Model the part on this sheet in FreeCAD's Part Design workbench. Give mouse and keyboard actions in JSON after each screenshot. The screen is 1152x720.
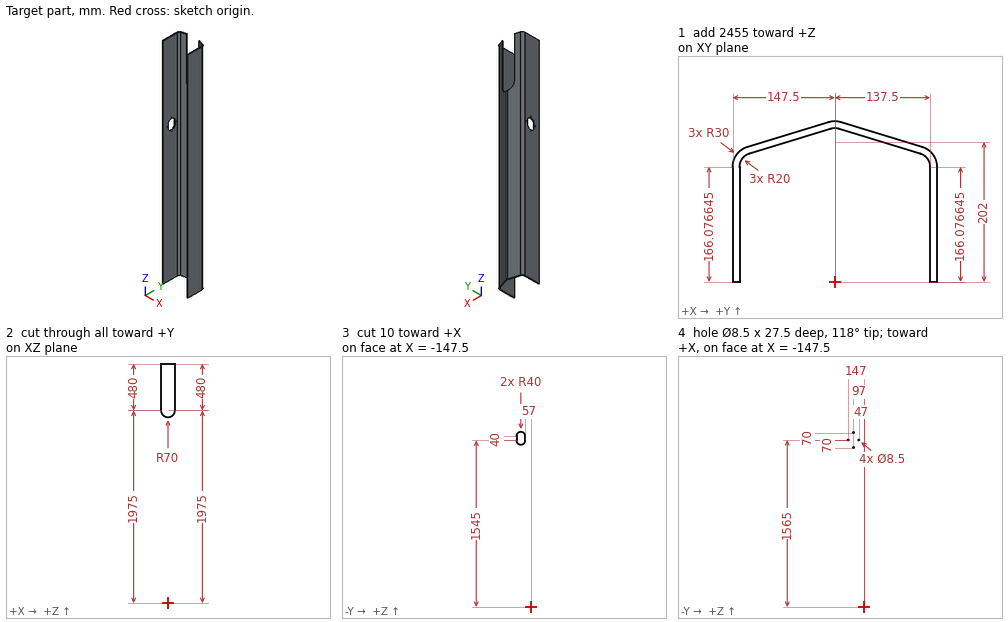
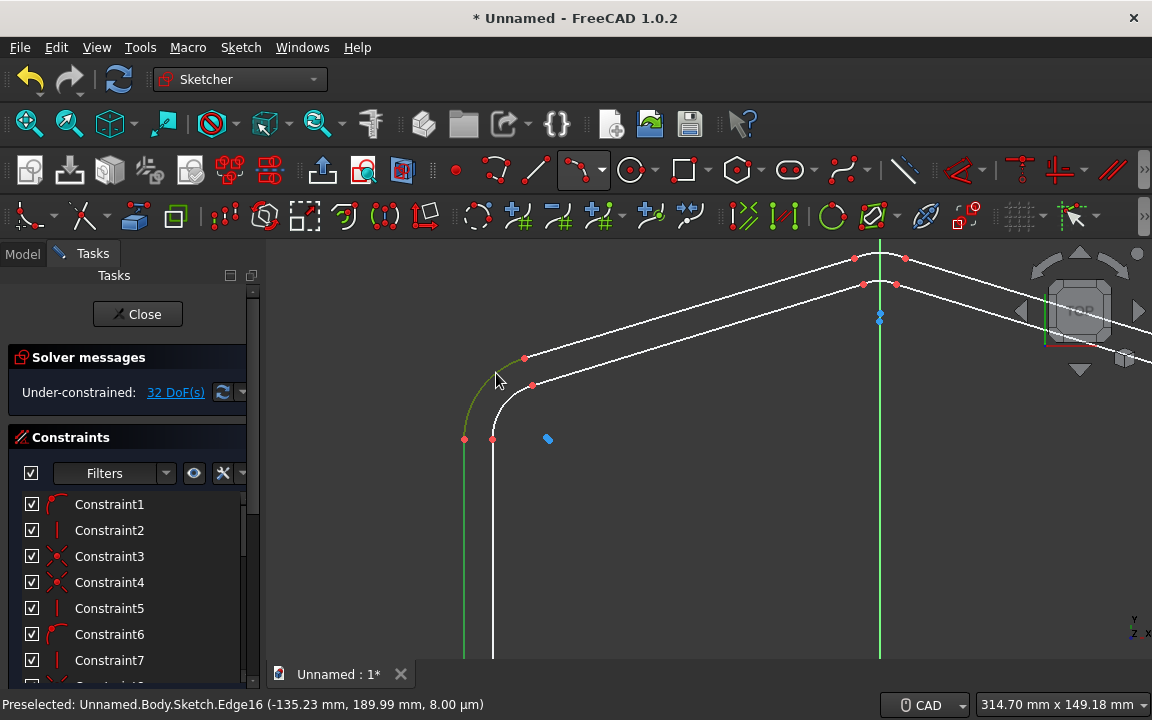
{"action": "key", "text": "t"}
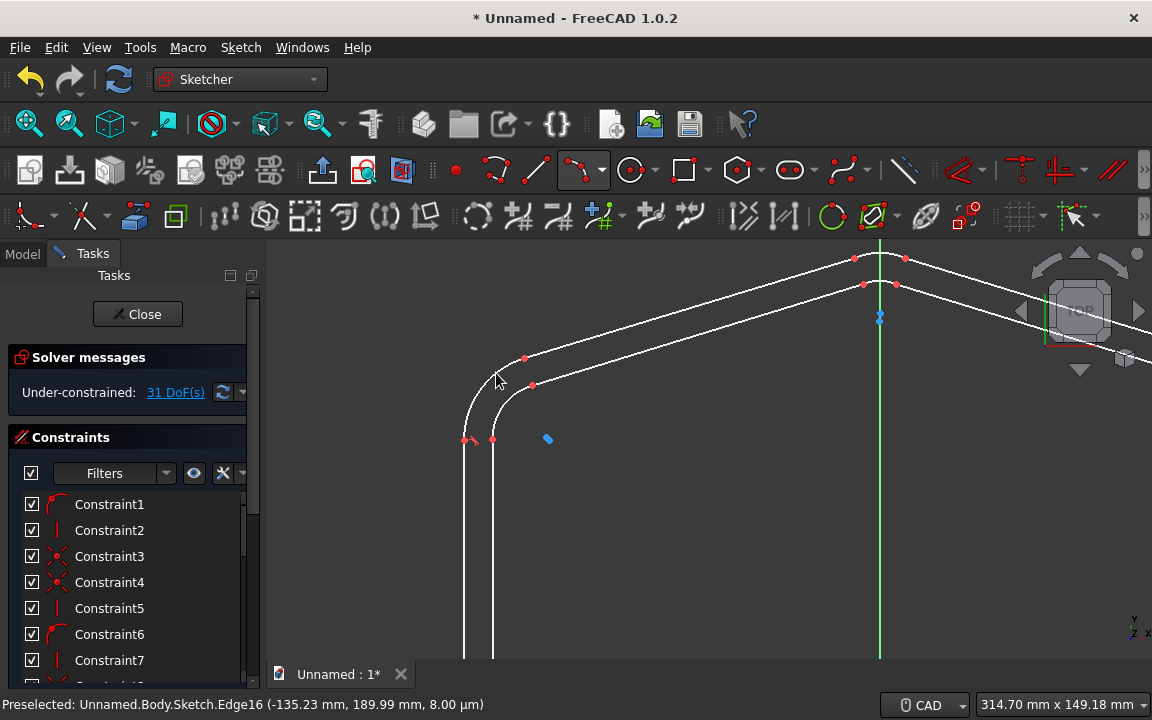
{"action": "left_click", "coordinate": [493, 576]}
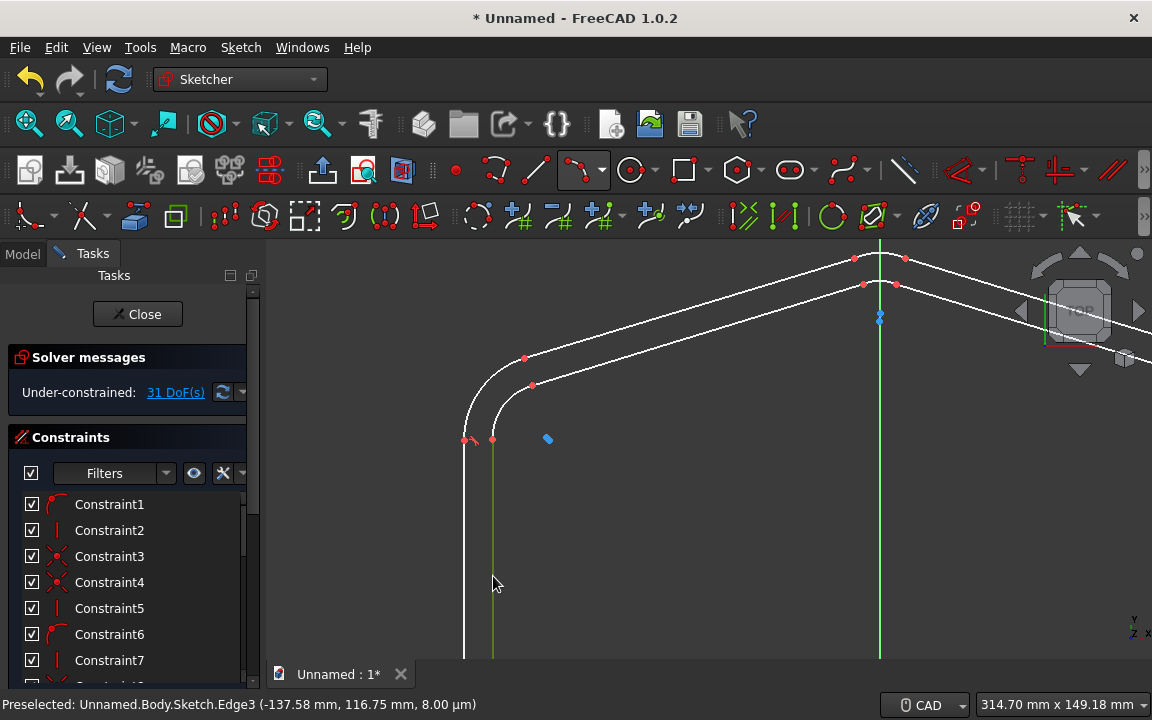
{"action": "left_click", "coordinate": [514, 395]}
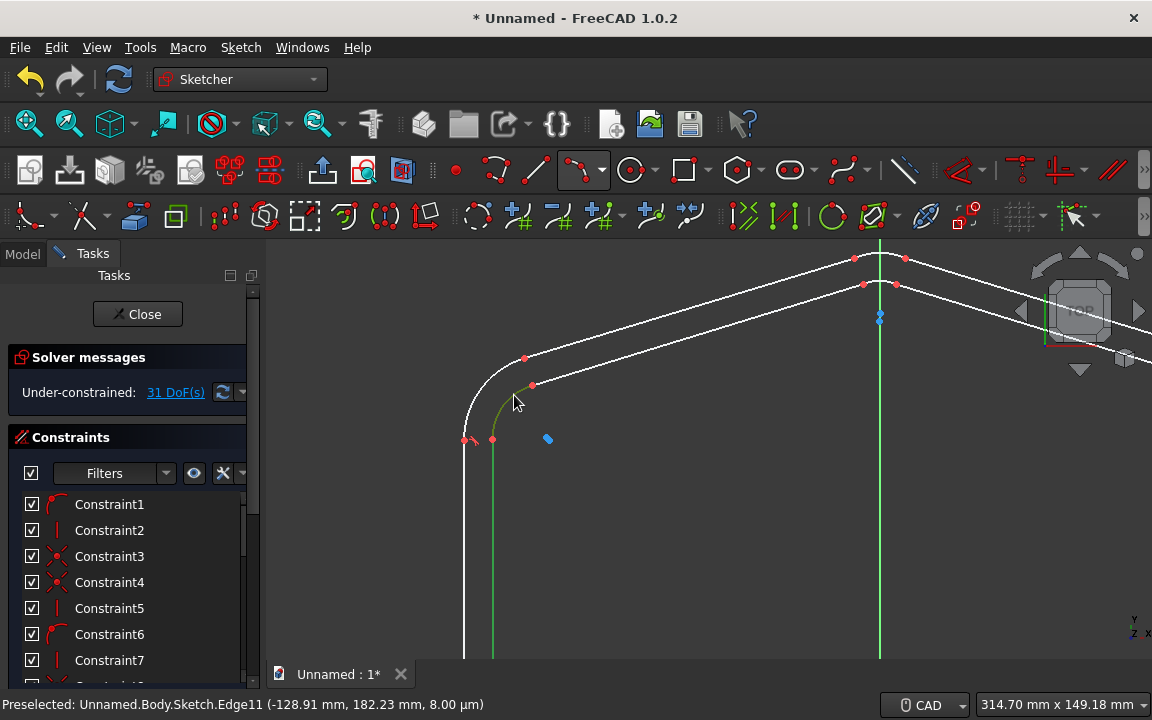
{"action": "key", "text": "t"}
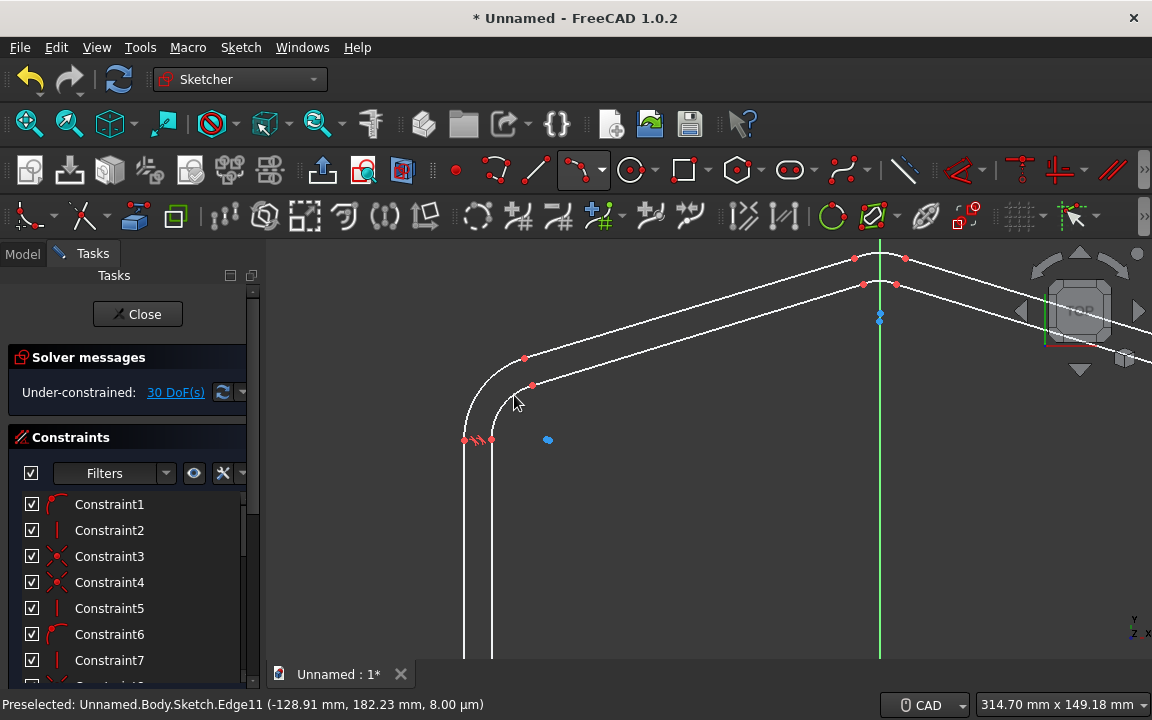
{"action": "left_click", "coordinate": [632, 355]}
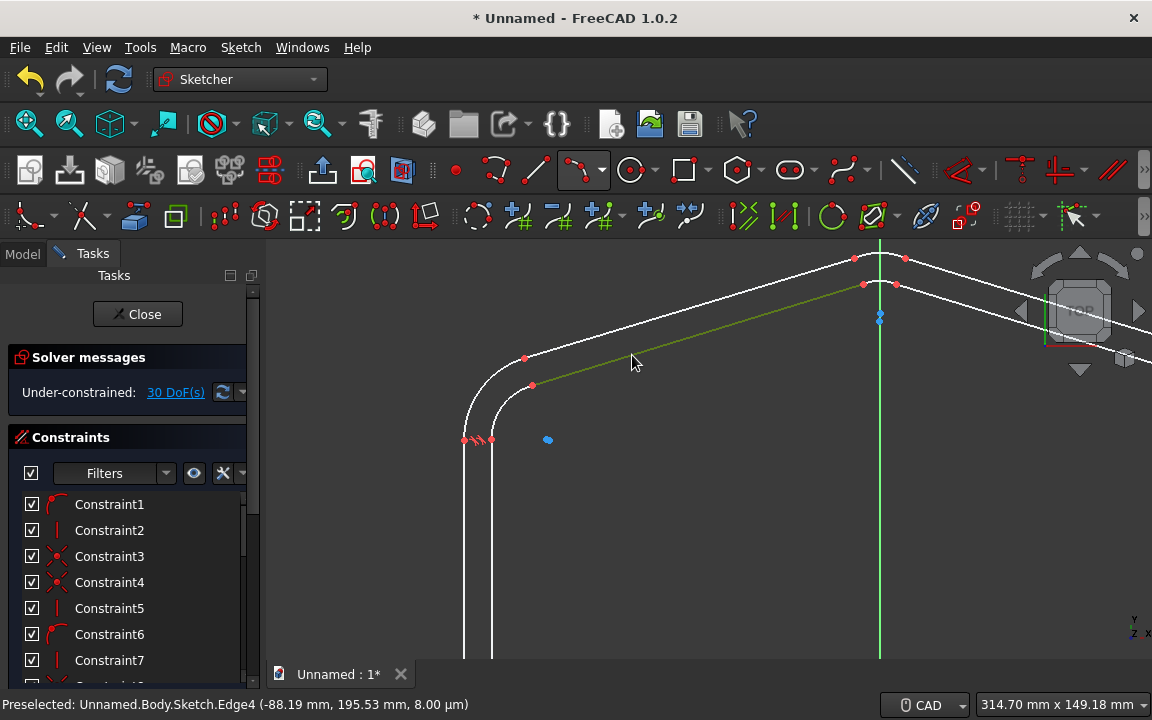
{"action": "left_click", "coordinate": [513, 395]}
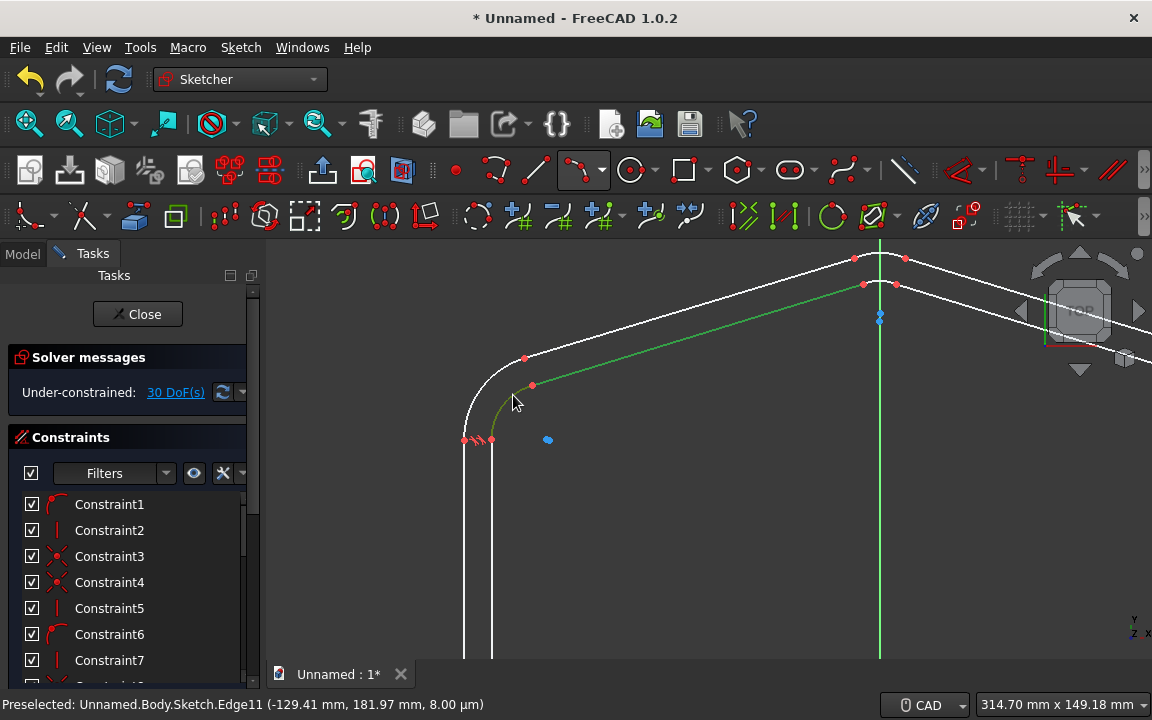
{"action": "key", "text": "t"}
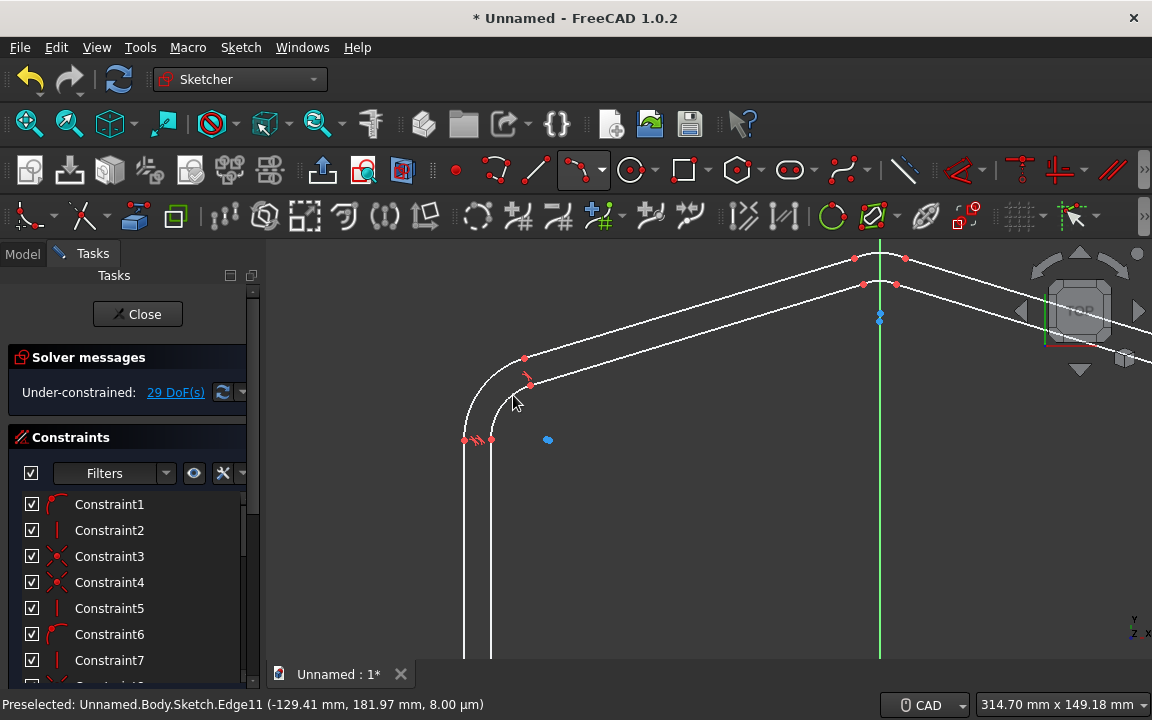
{"action": "left_click", "coordinate": [630, 355]}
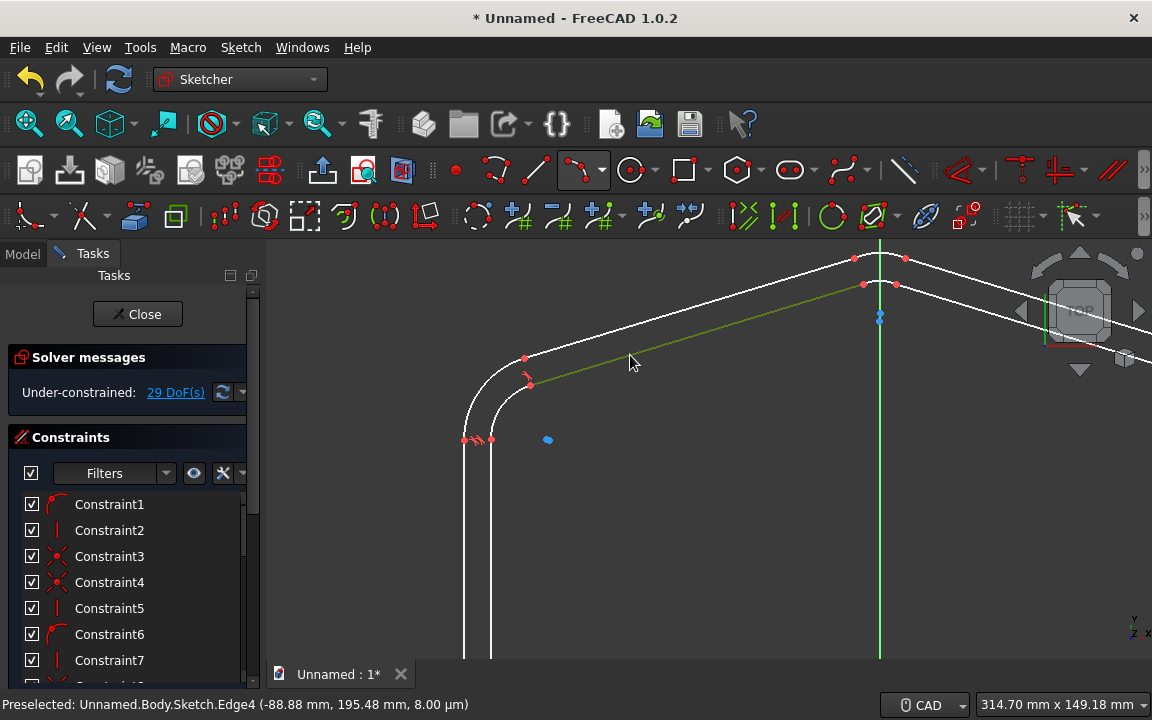
{"action": "left_click", "coordinate": [880, 281]}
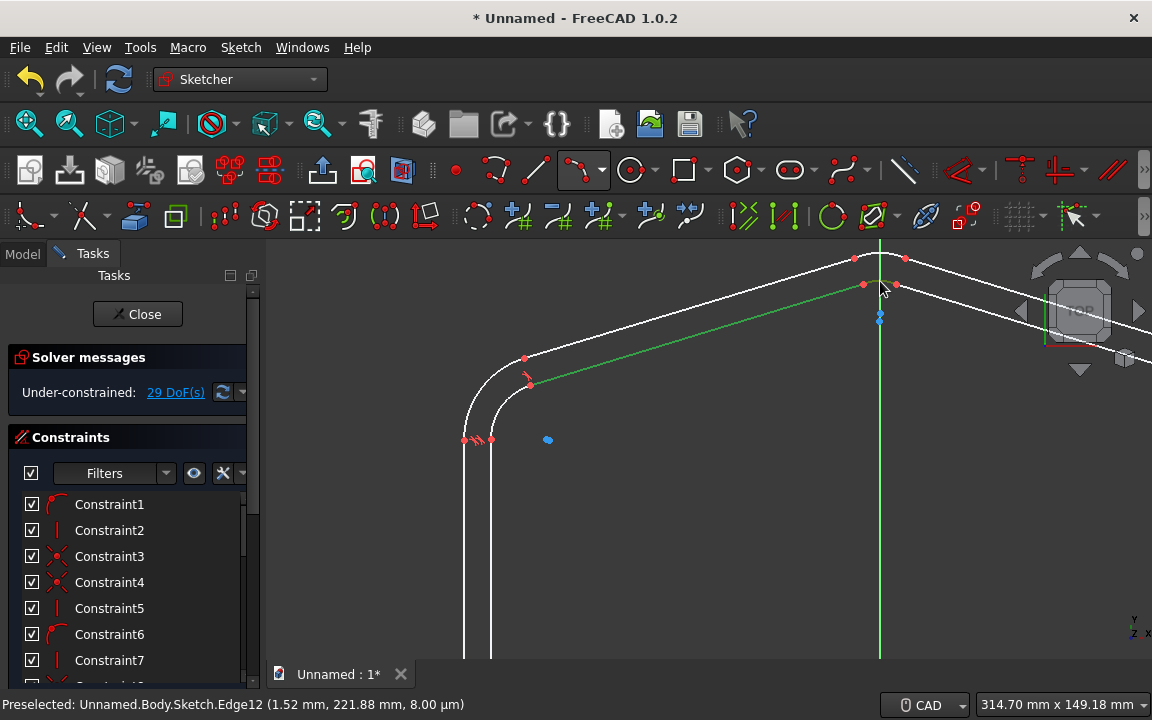
{"action": "key", "text": "t"}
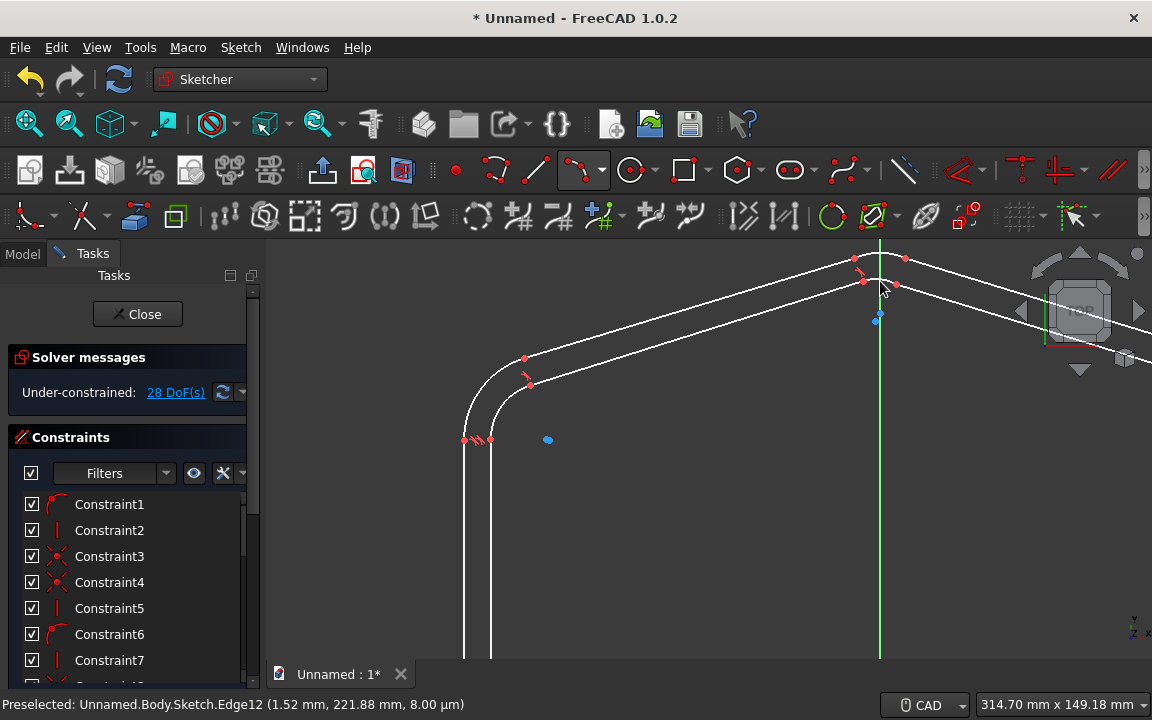
{"action": "left_click", "coordinate": [962, 305]}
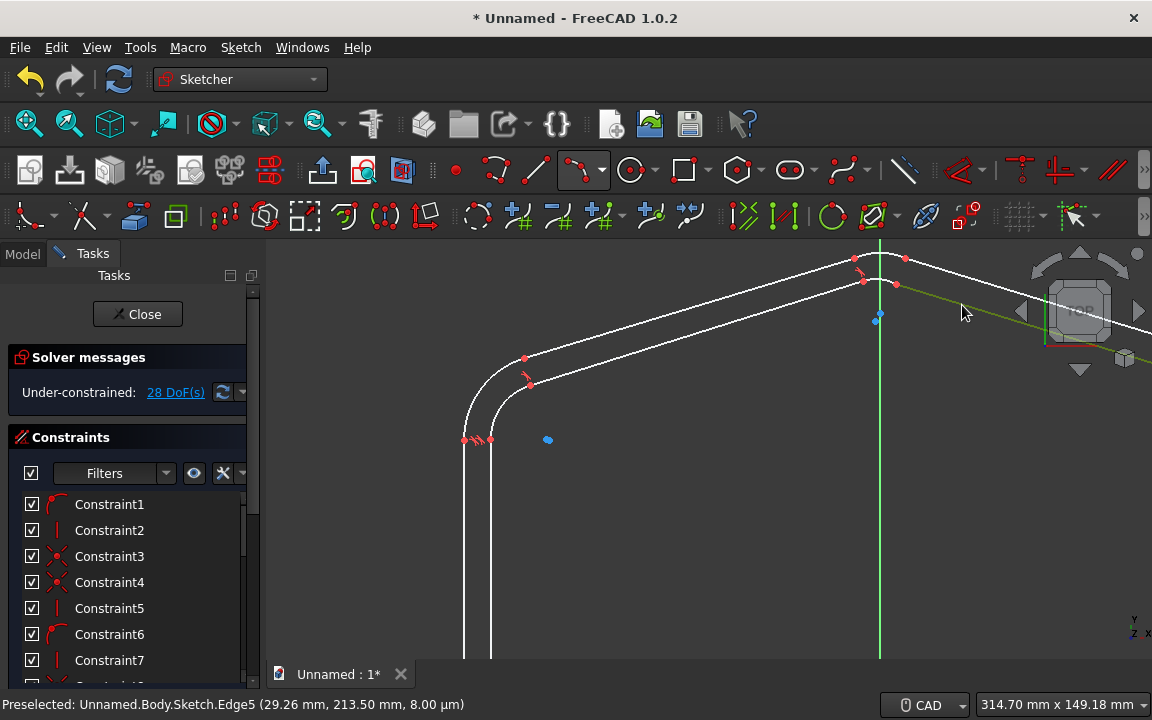
{"action": "left_click", "coordinate": [880, 279]}